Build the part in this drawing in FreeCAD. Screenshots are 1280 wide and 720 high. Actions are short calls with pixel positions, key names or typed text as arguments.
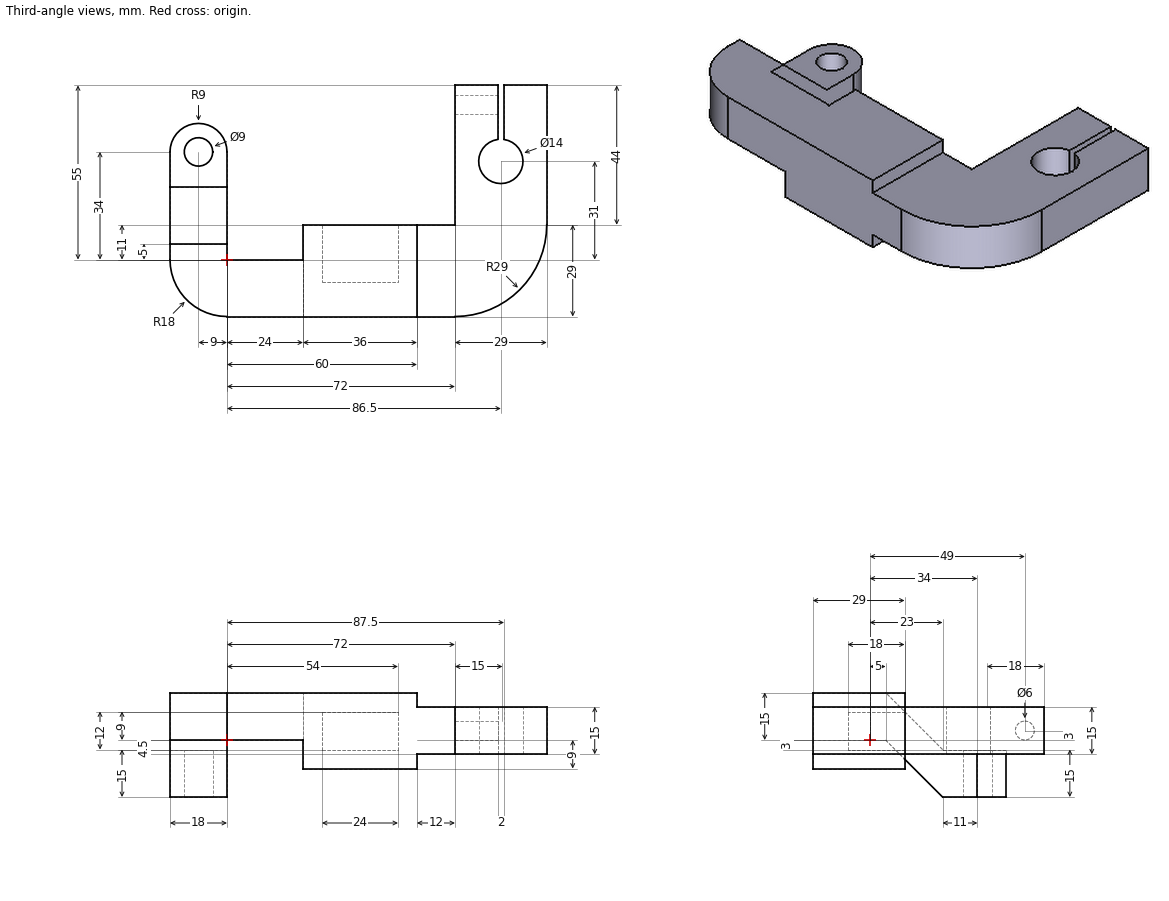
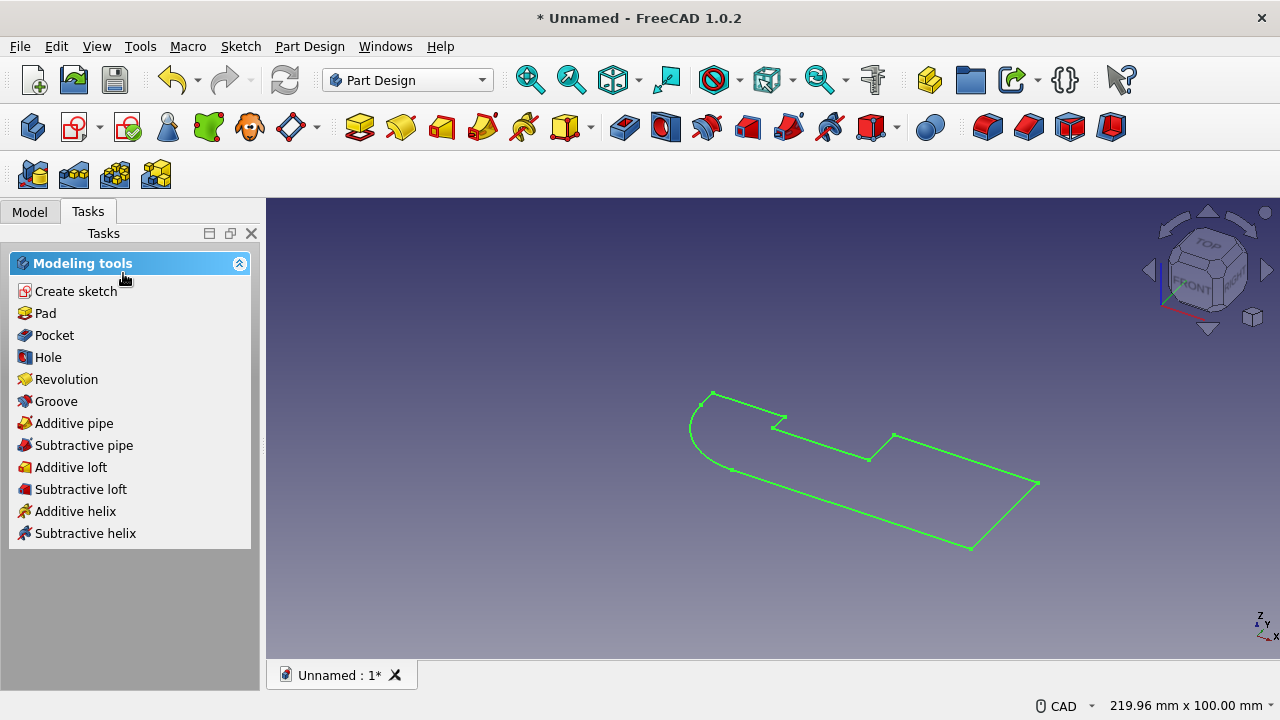
click(360, 128)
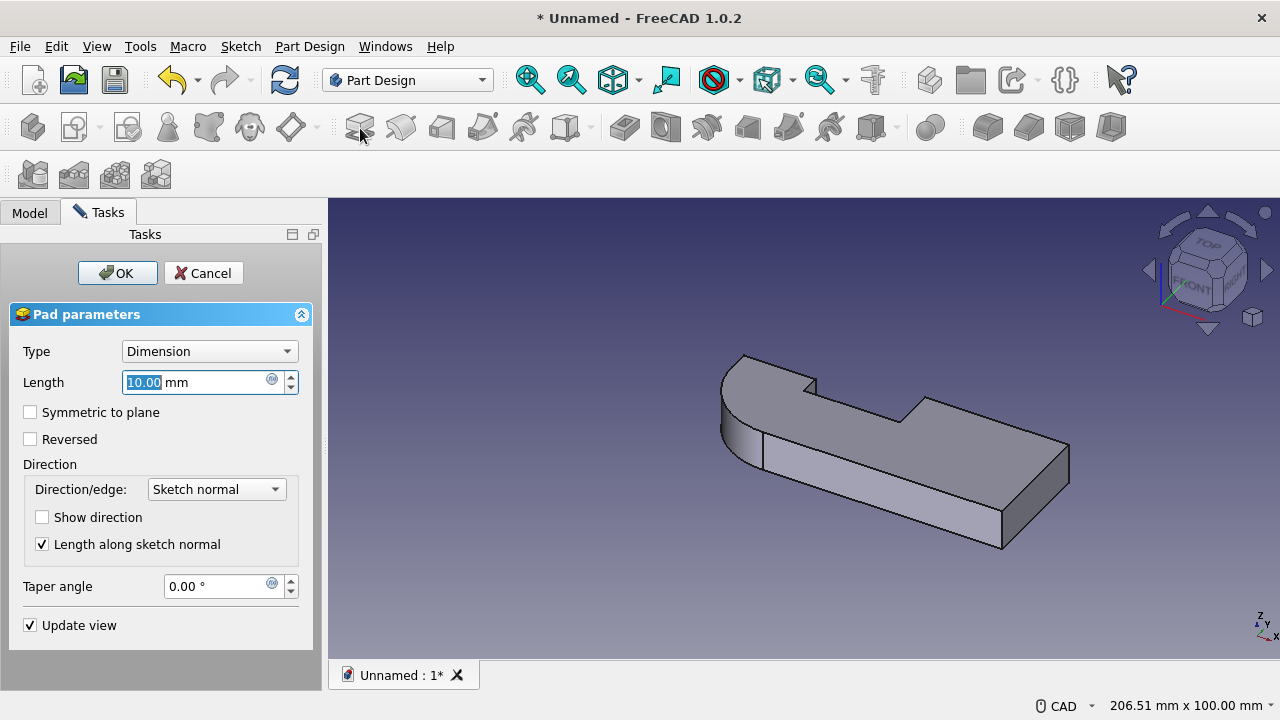
text(15)
key(Tab)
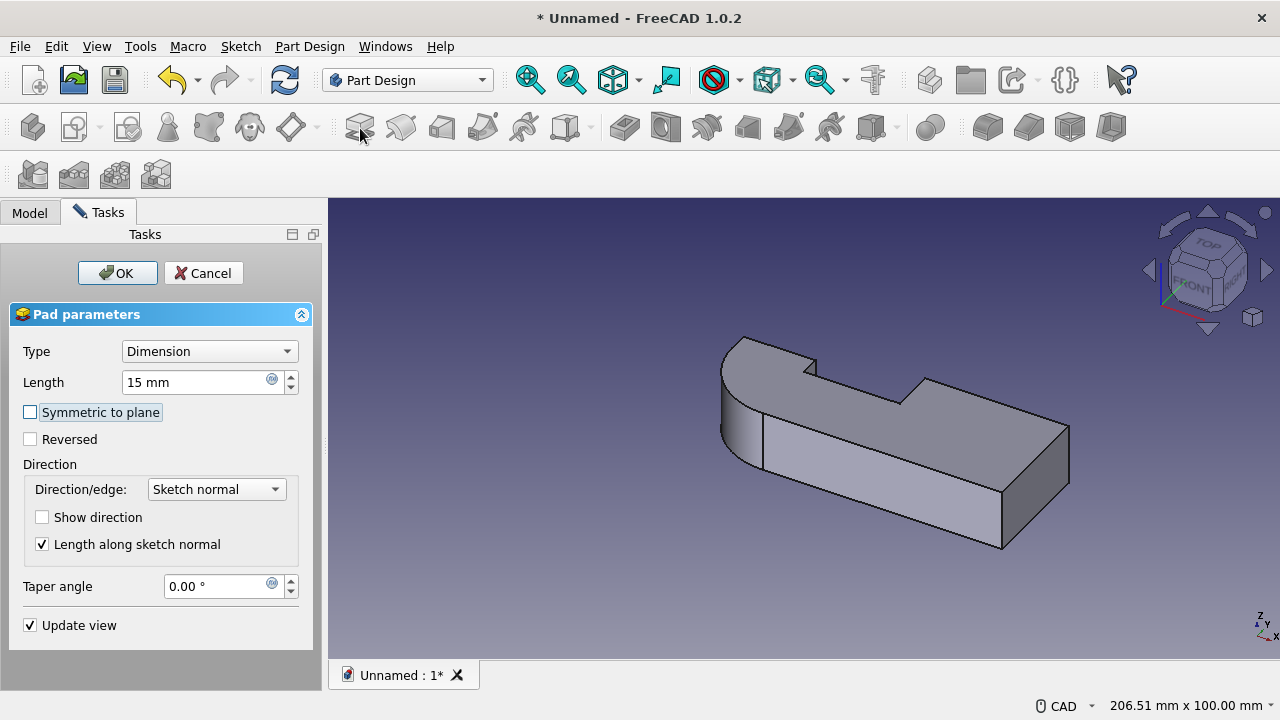
click(118, 273)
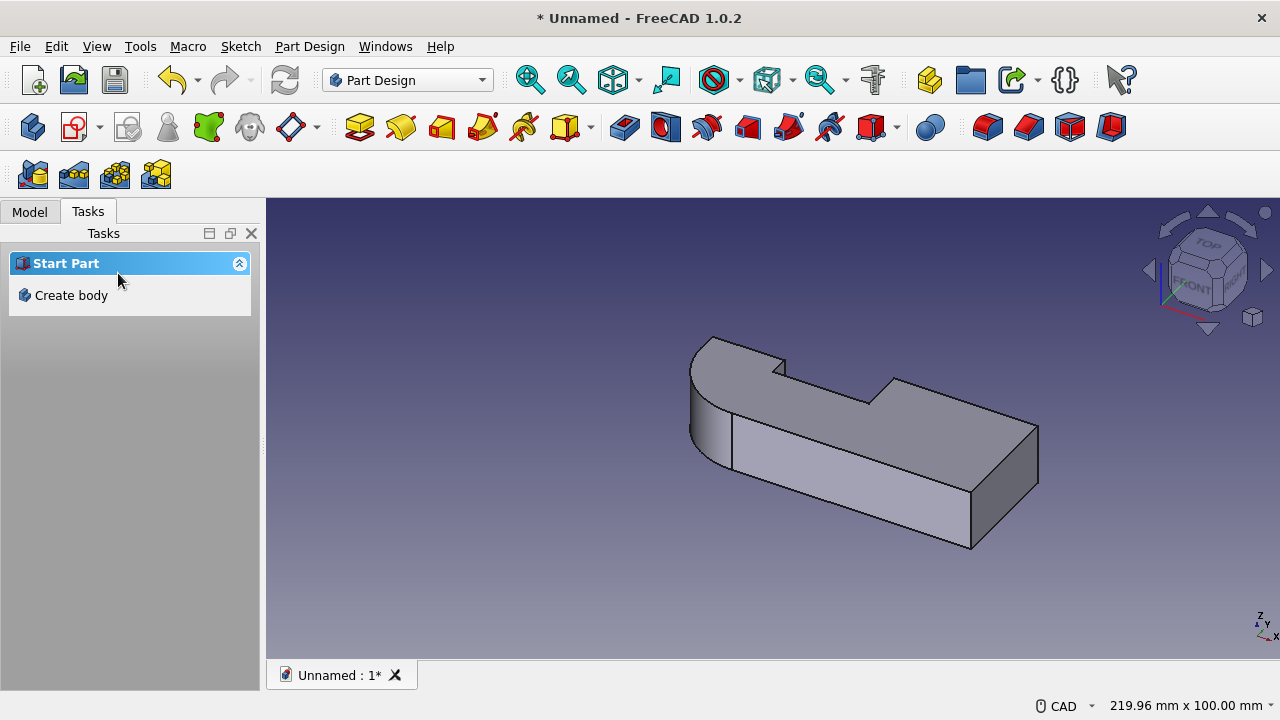
key(6)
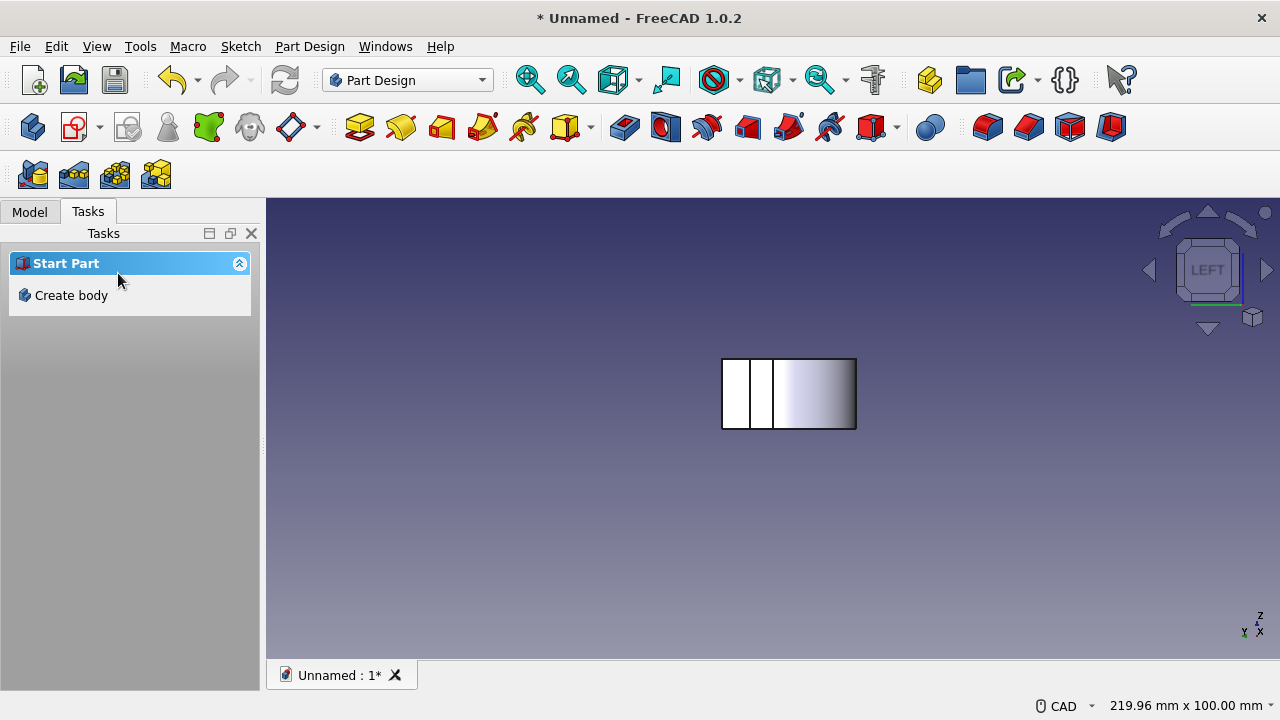
click(531, 80)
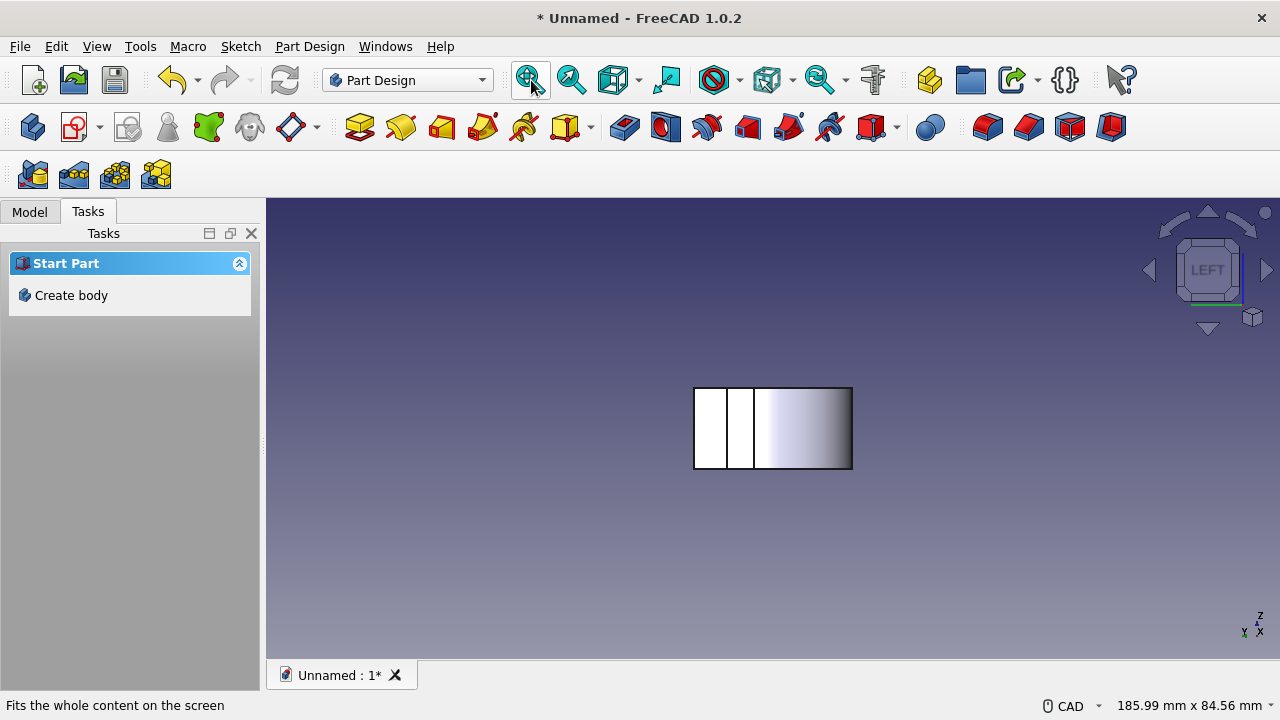
click(740, 404)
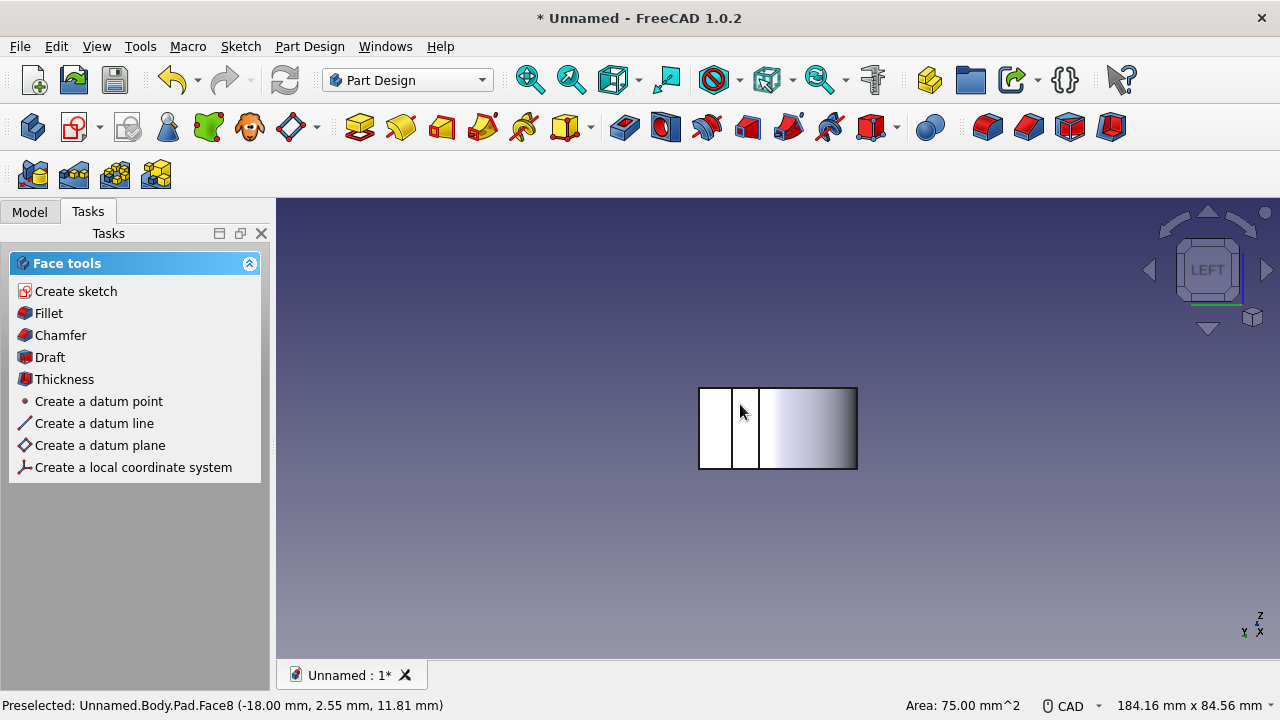
click(74, 128)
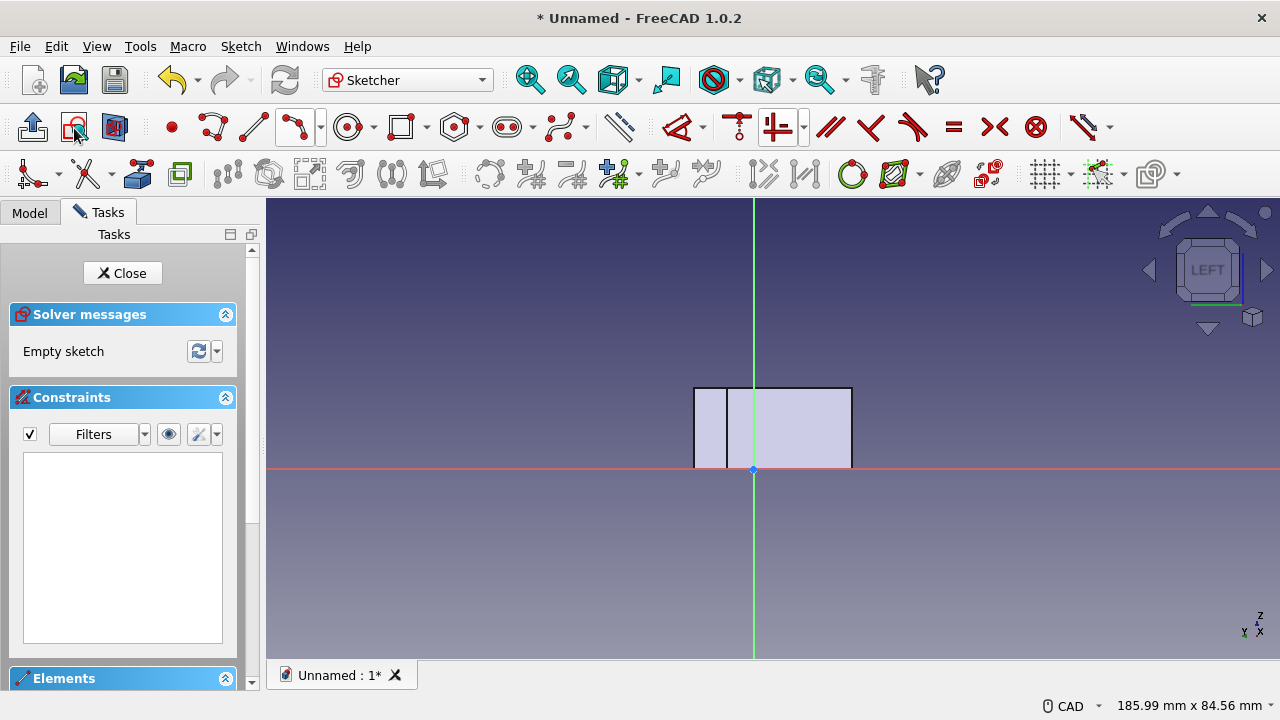
scroll(664, 577, up, 2)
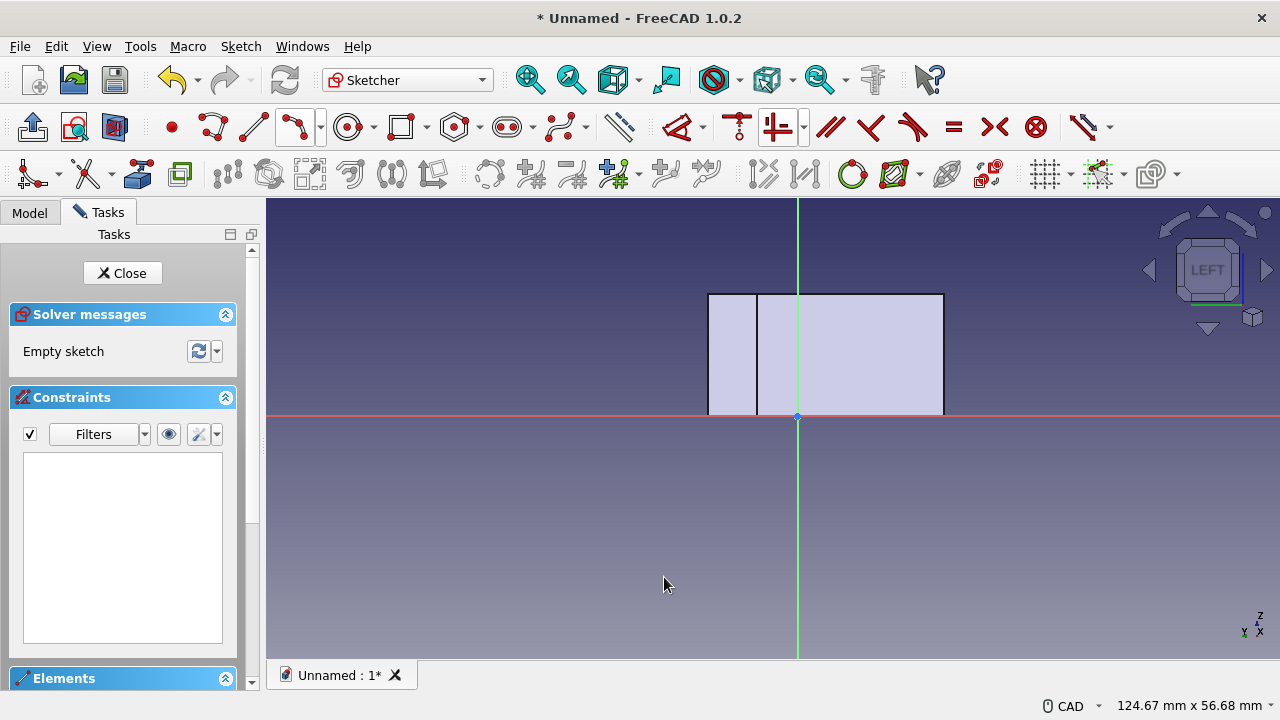
click(213, 128)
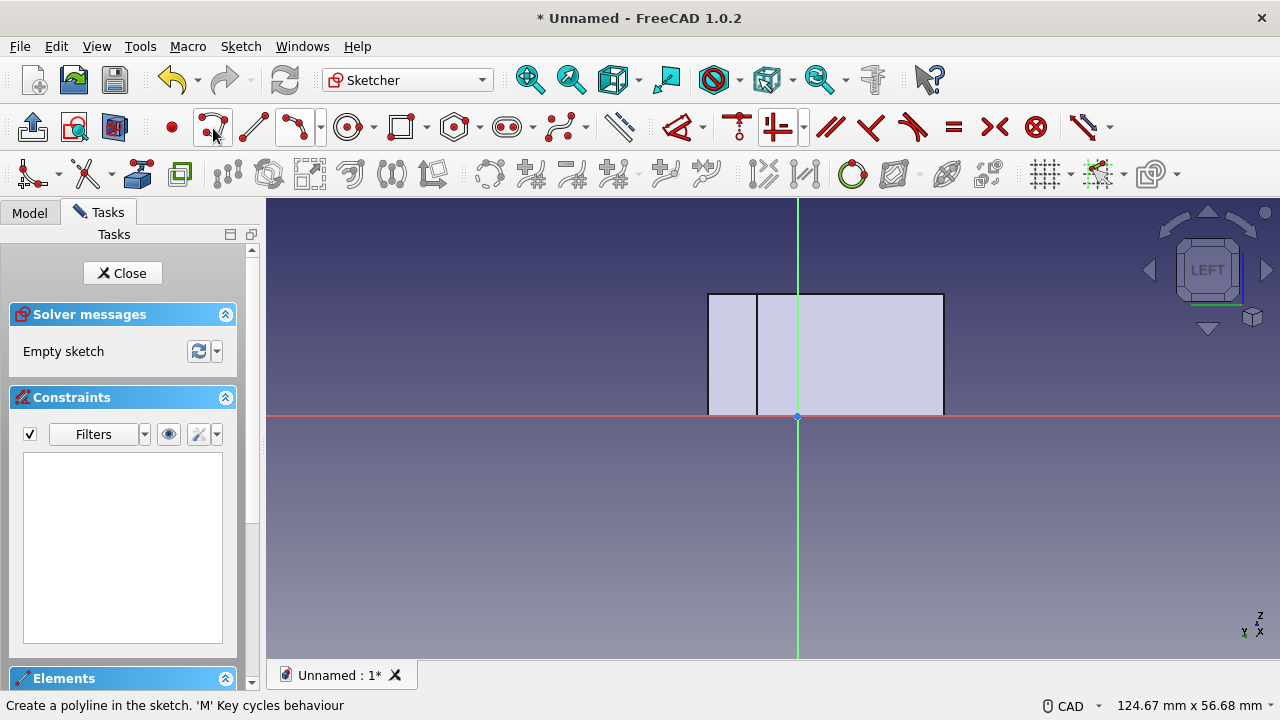
click(757, 416)
click(757, 294)
click(611, 440)
click(611, 562)
click(757, 416)
key(Escape)
key(Escape)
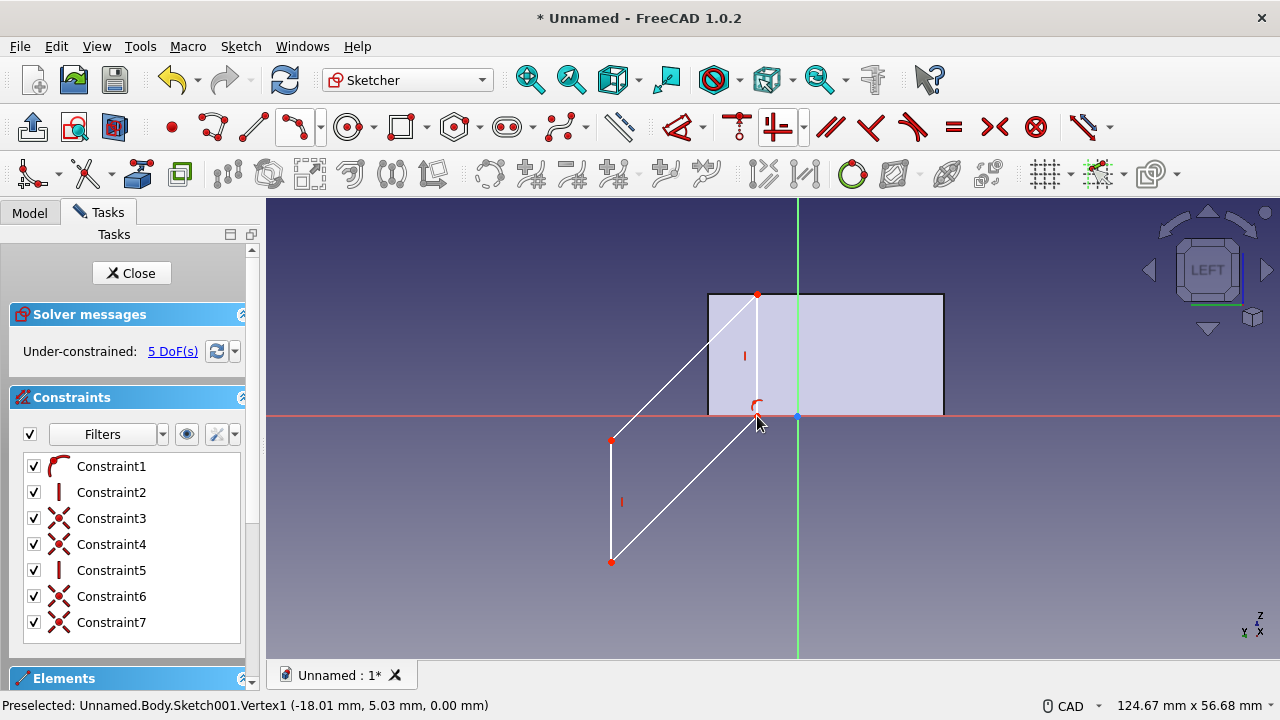
click(676, 128)